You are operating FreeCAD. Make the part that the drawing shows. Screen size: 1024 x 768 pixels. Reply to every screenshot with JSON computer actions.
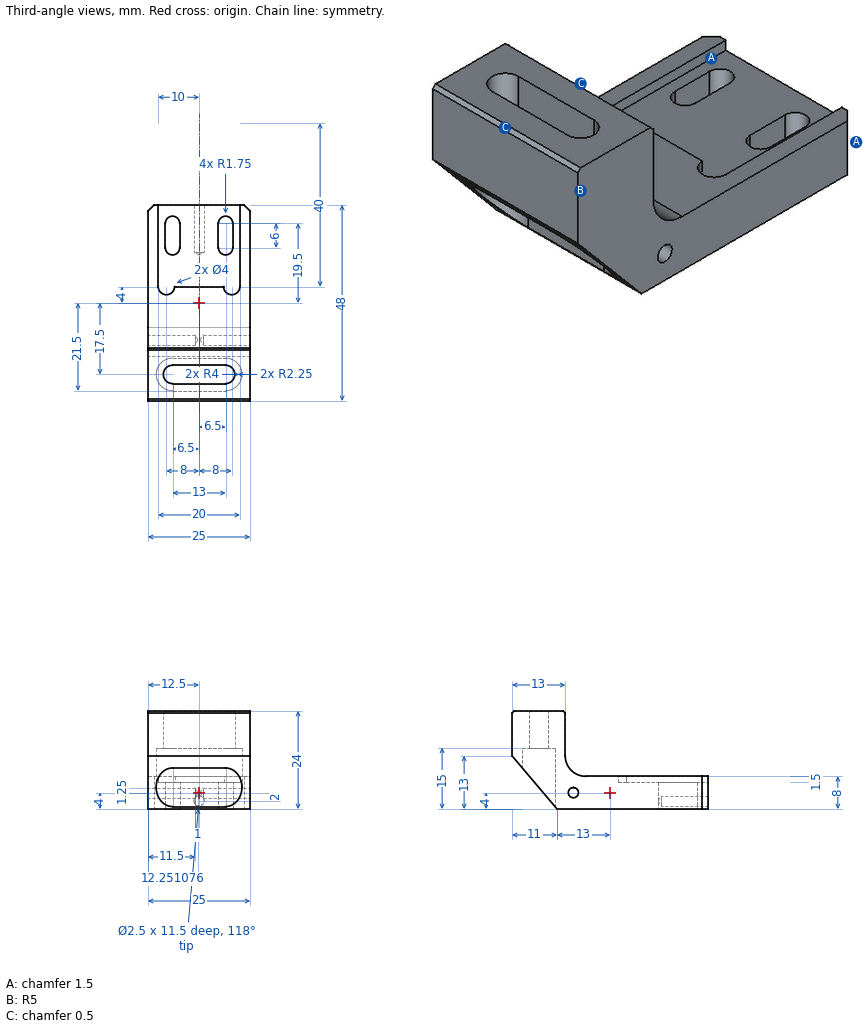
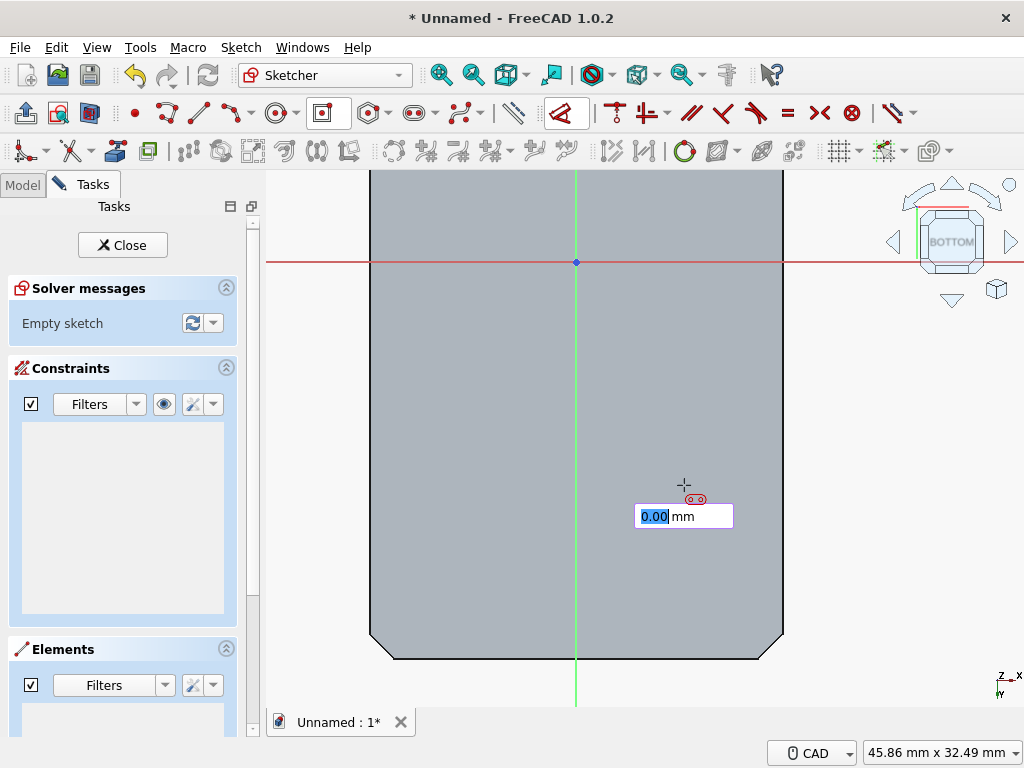
{"action": "left_click", "coordinate": [655, 535]}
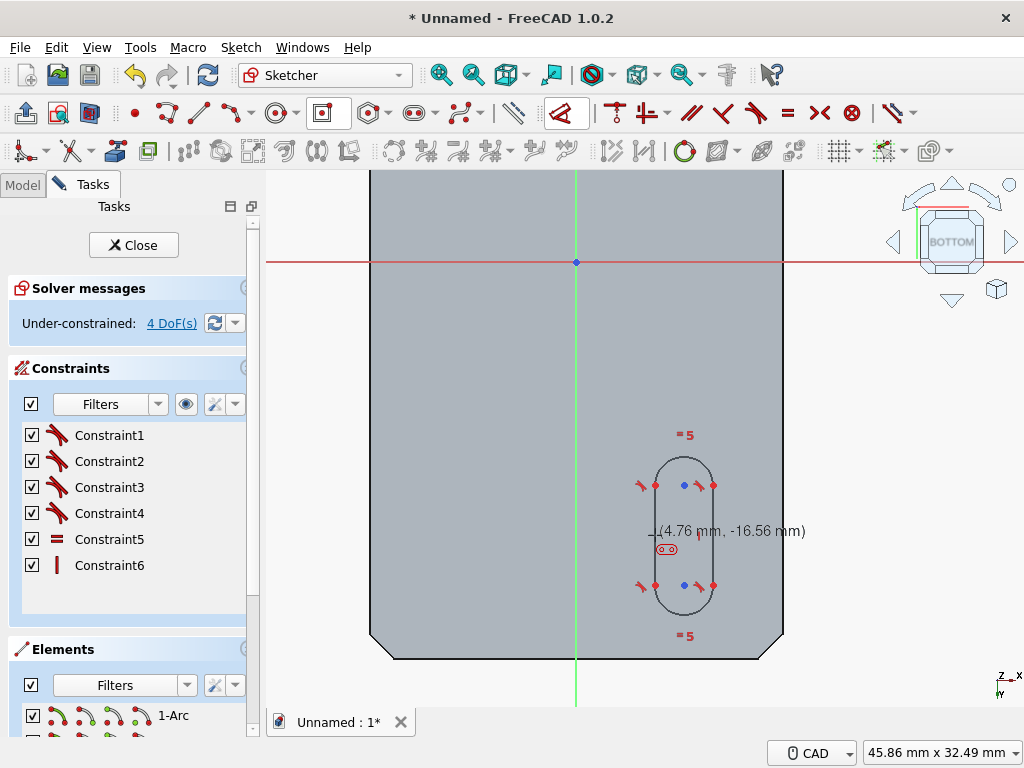
{"action": "left_click", "coordinate": [469, 585]}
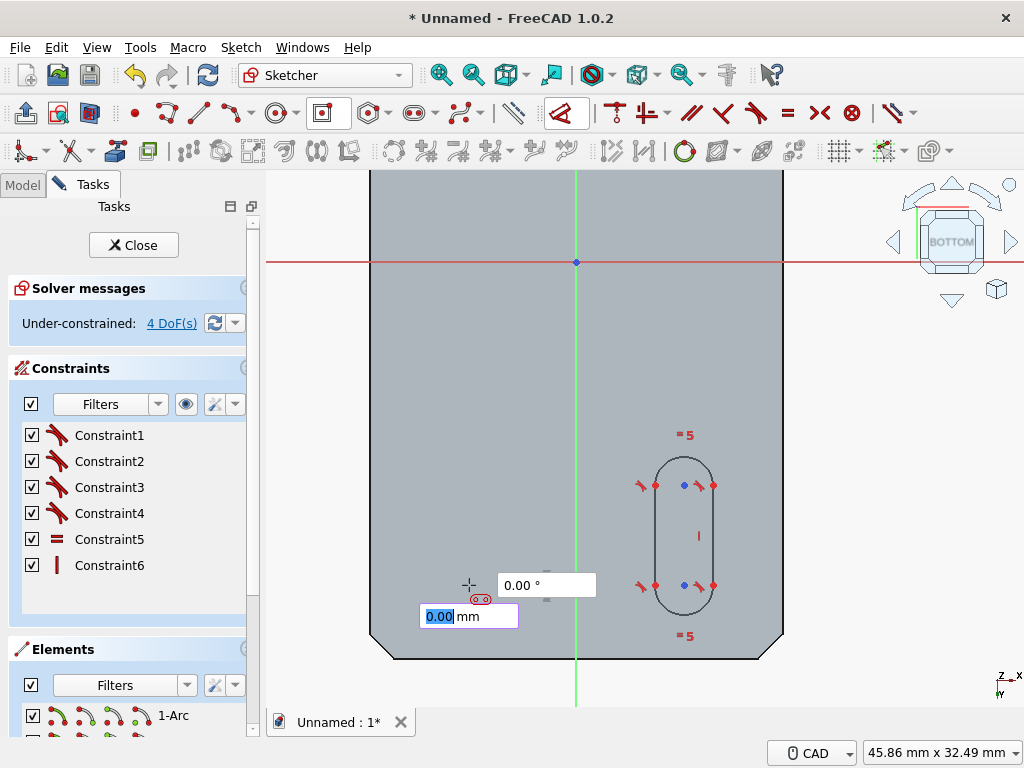
{"action": "left_click", "coordinate": [469, 485]}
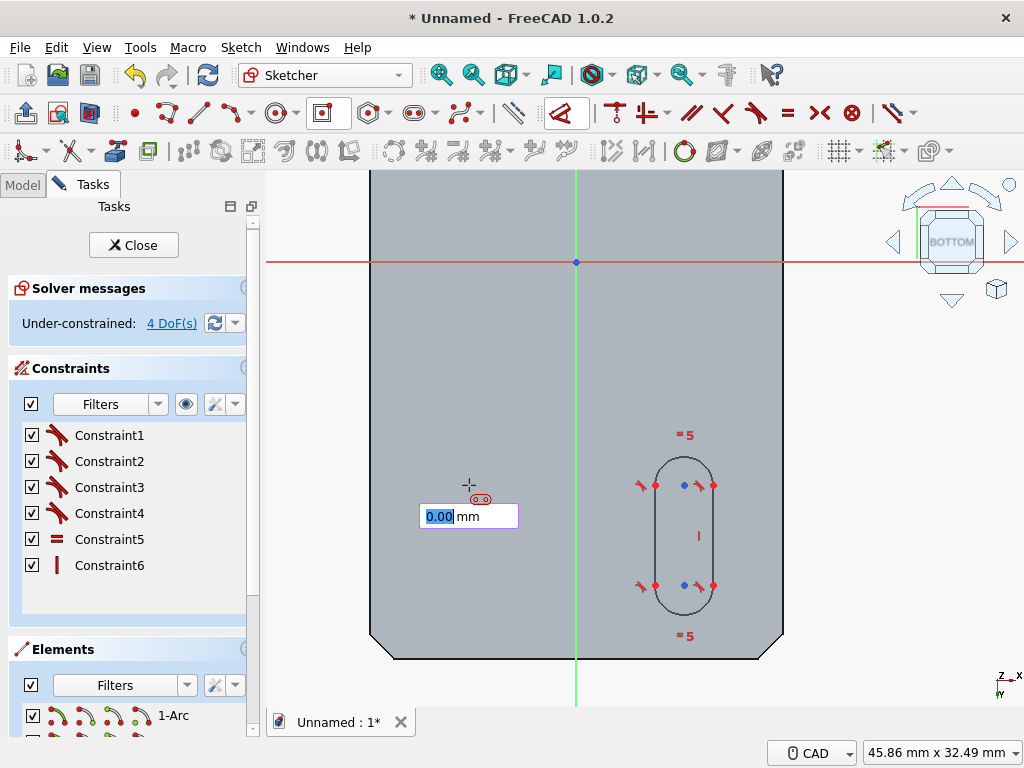
{"action": "left_click", "coordinate": [440, 535]}
{"action": "key", "text": "Escape"}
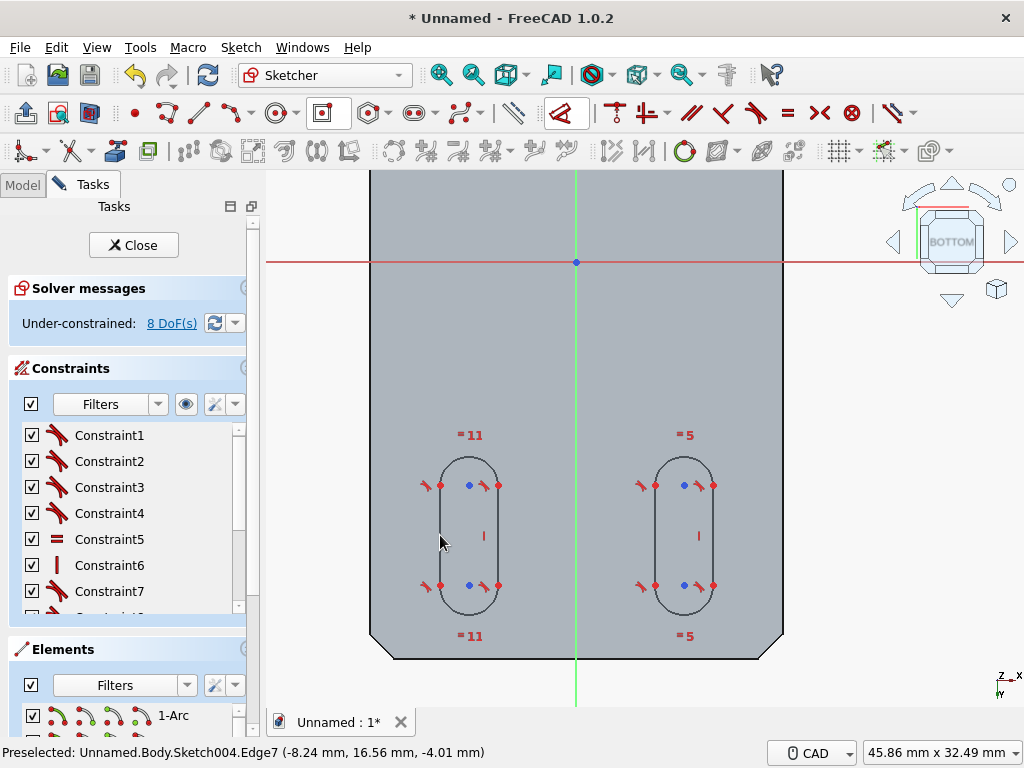
{"action": "left_click", "coordinate": [667, 609]}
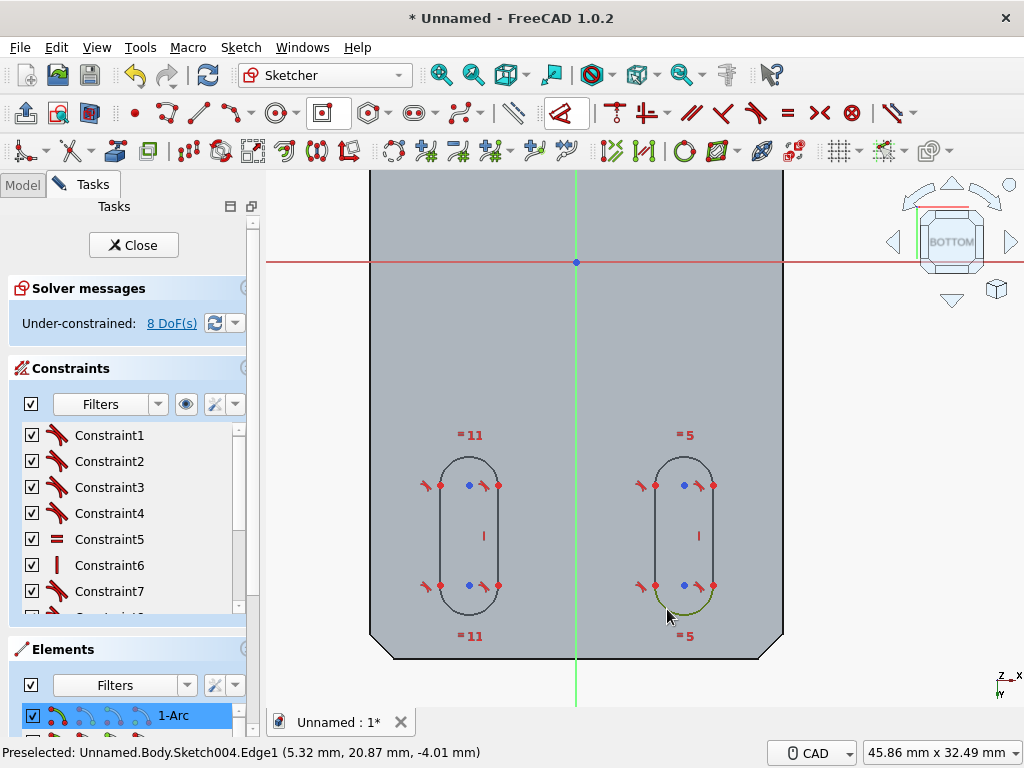
{"action": "left_click", "coordinate": [452, 609]}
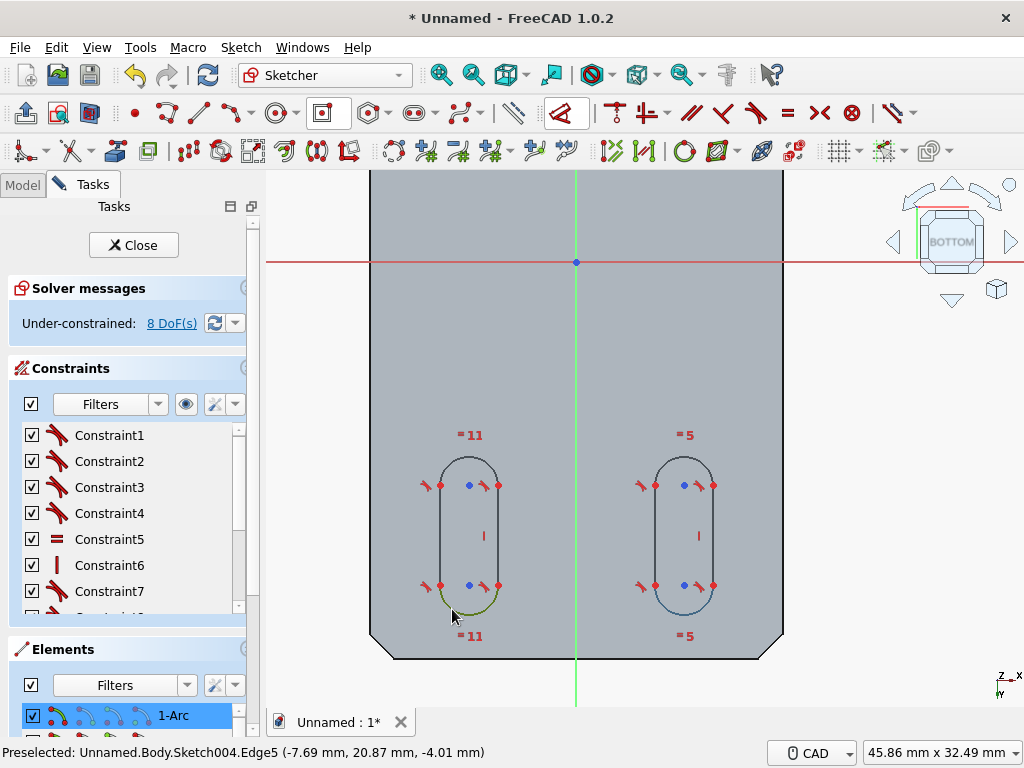
{"action": "left_click", "coordinate": [788, 114]}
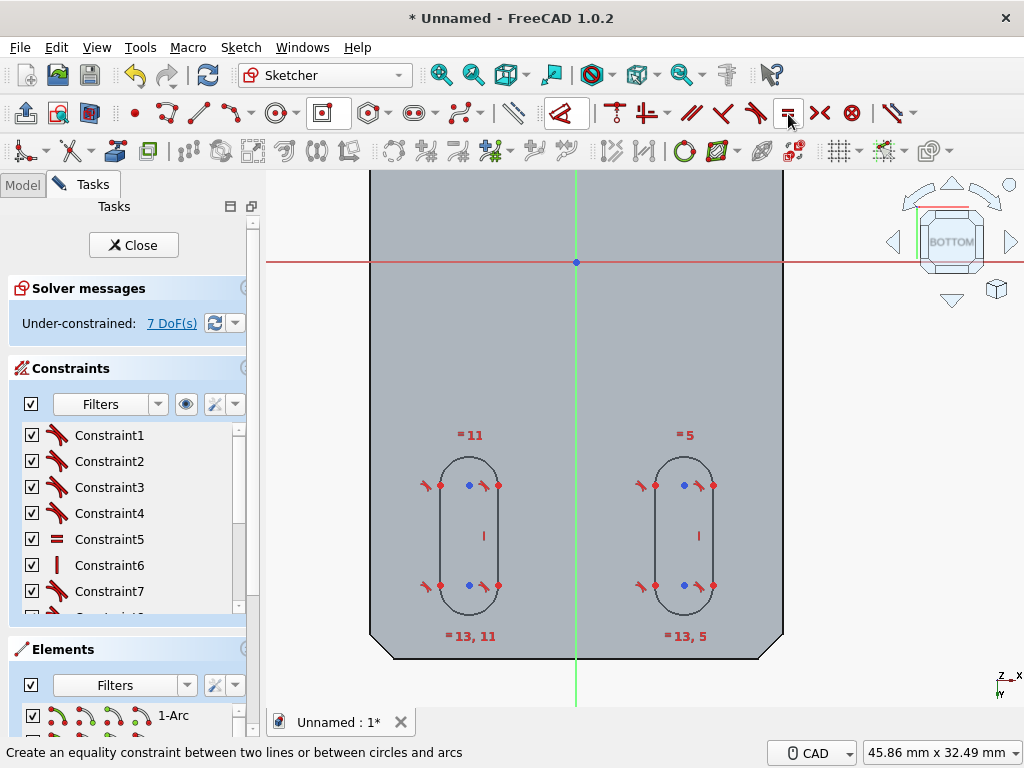
{"action": "left_click", "coordinate": [684, 586]}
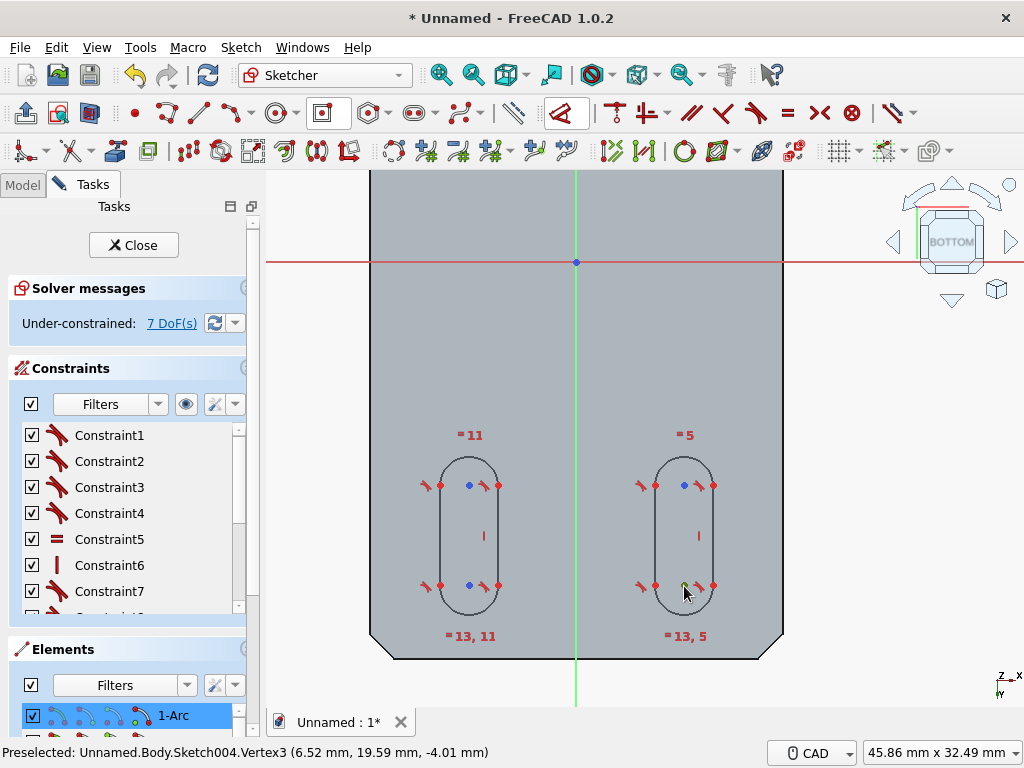
{"action": "left_click", "coordinate": [469, 586]}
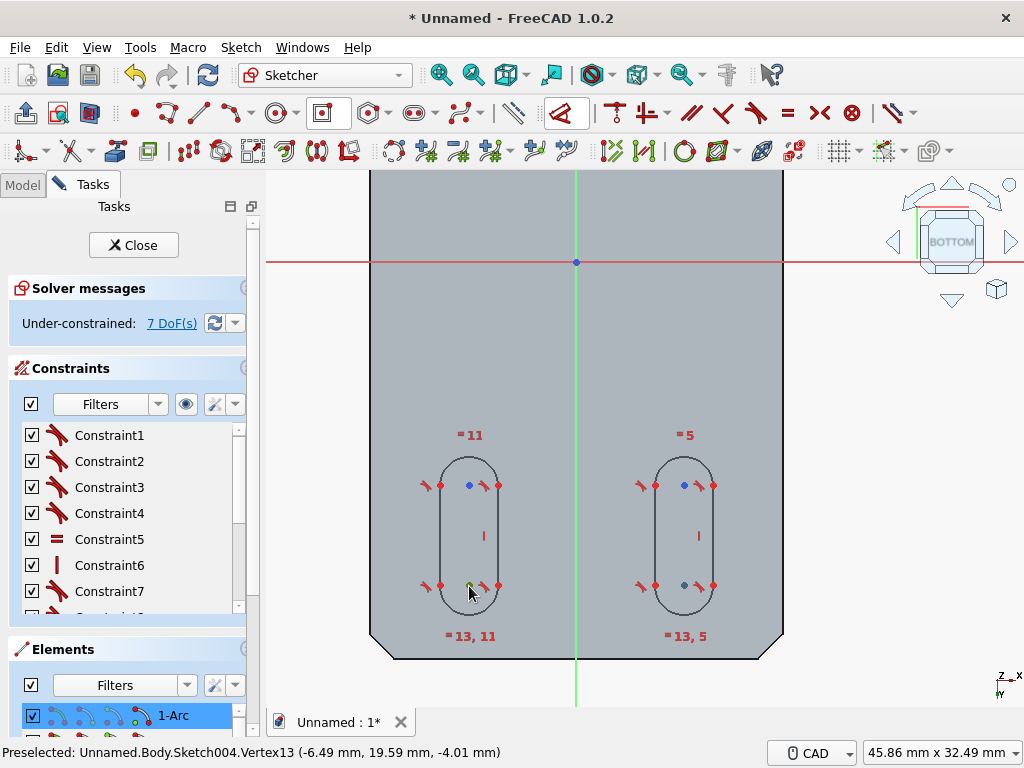
{"action": "left_click", "coordinate": [576, 645]}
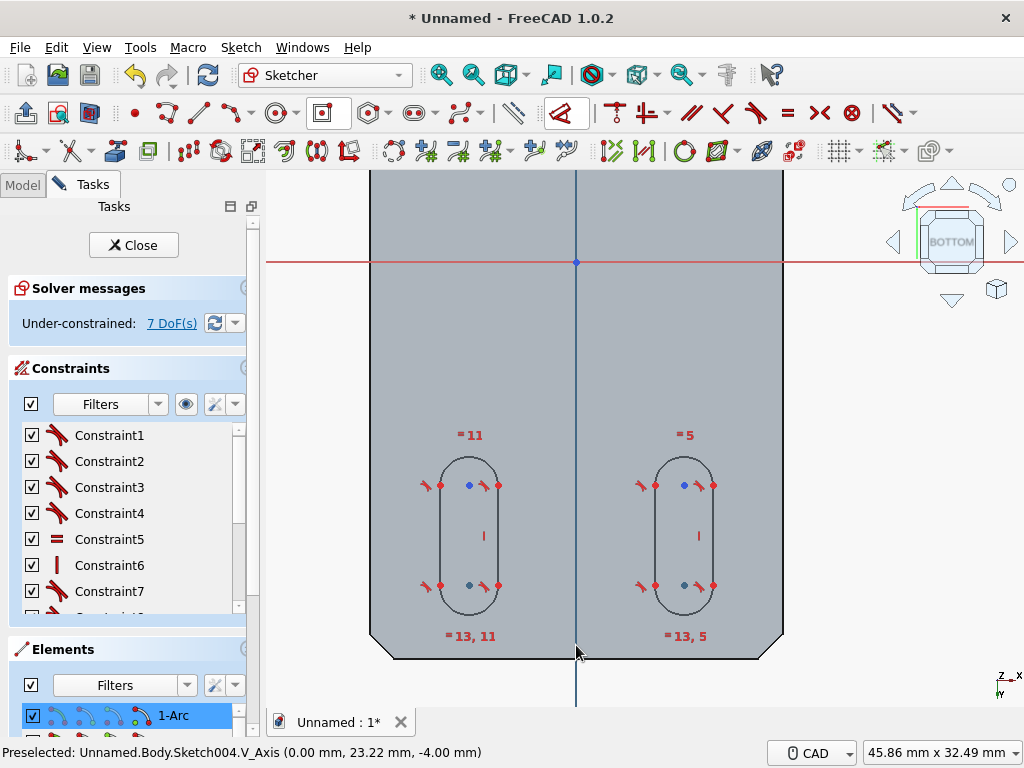
{"action": "left_click", "coordinate": [820, 114]}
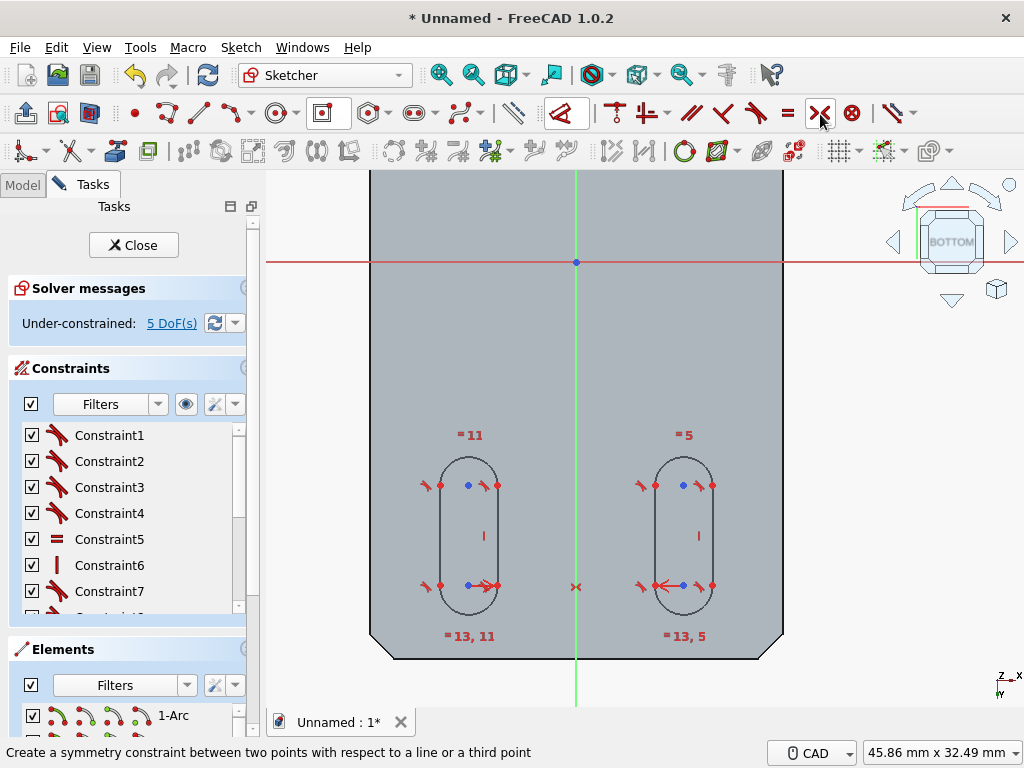
{"action": "scroll", "coordinate": [667, 609], "scroll_direction": "up", "scroll_amount": 2}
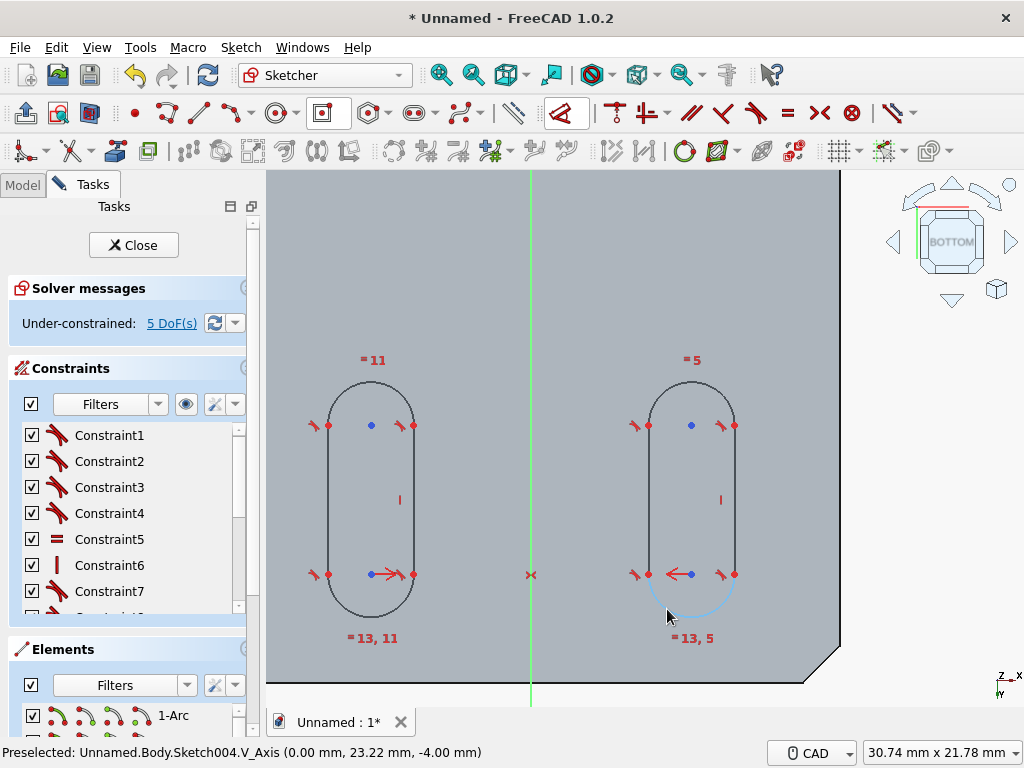
{"action": "left_click", "coordinate": [667, 609]}